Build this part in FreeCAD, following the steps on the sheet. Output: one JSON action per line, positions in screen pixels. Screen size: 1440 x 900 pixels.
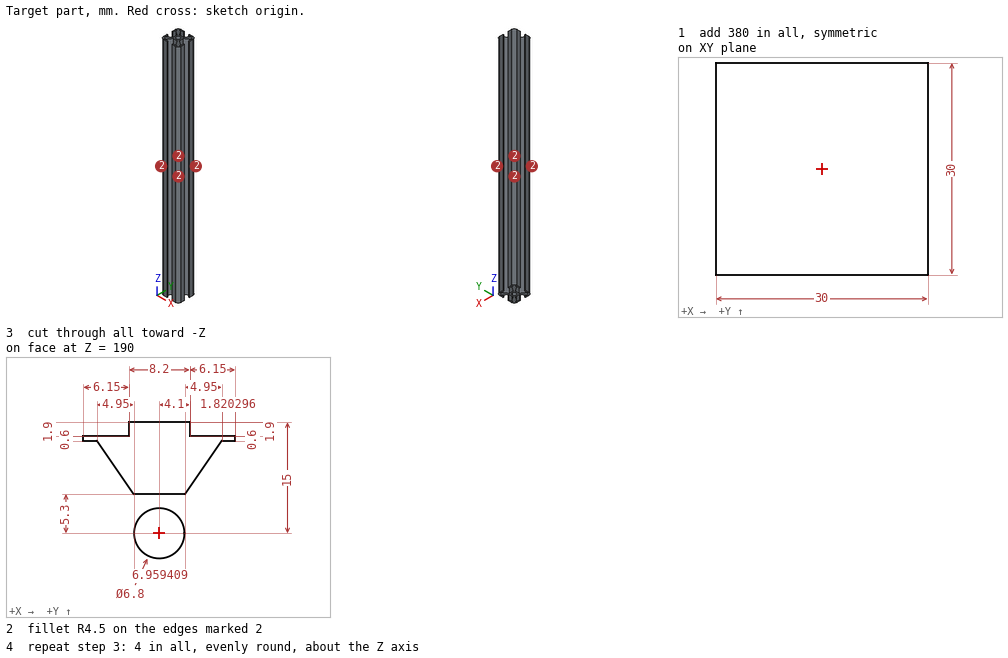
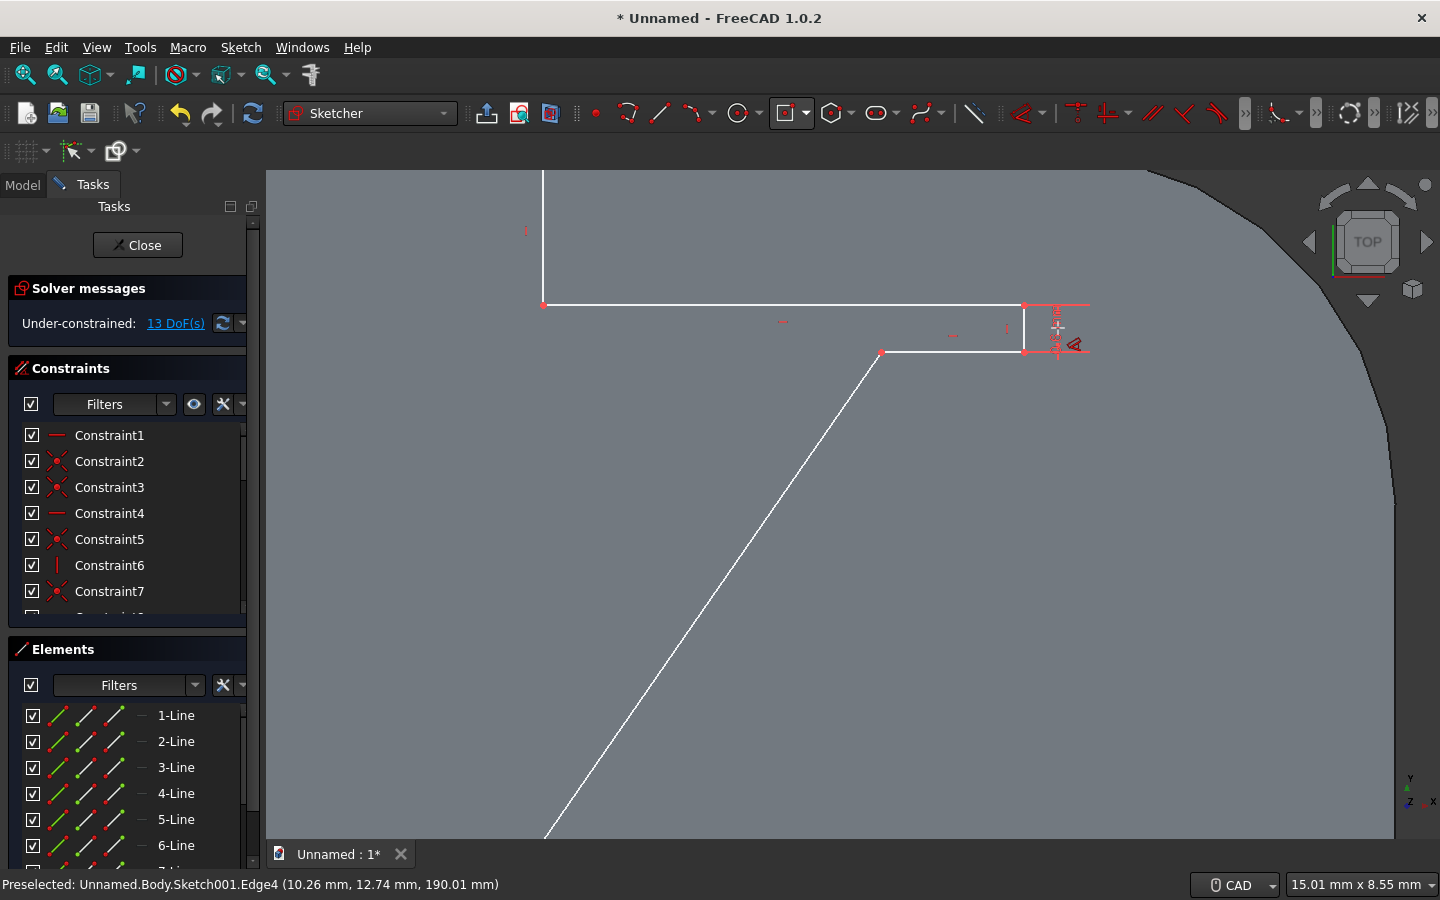
{"action": "left_click", "coordinate": [543, 260]}
{"action": "left_click", "coordinate": [577, 252]}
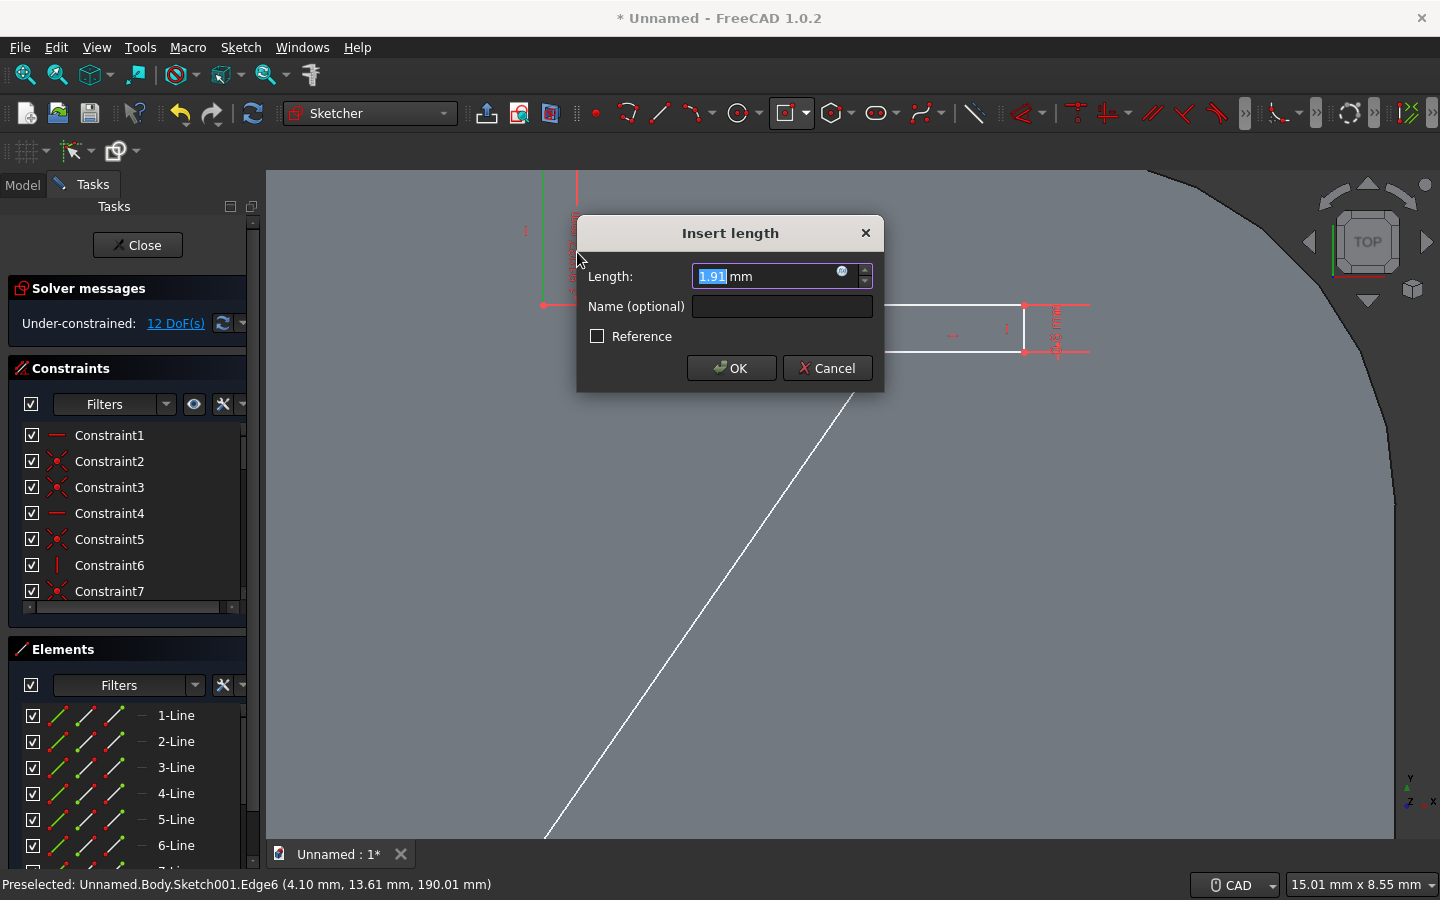
{"action": "type", "text": "1.9"}
{"action": "key", "text": "Return"}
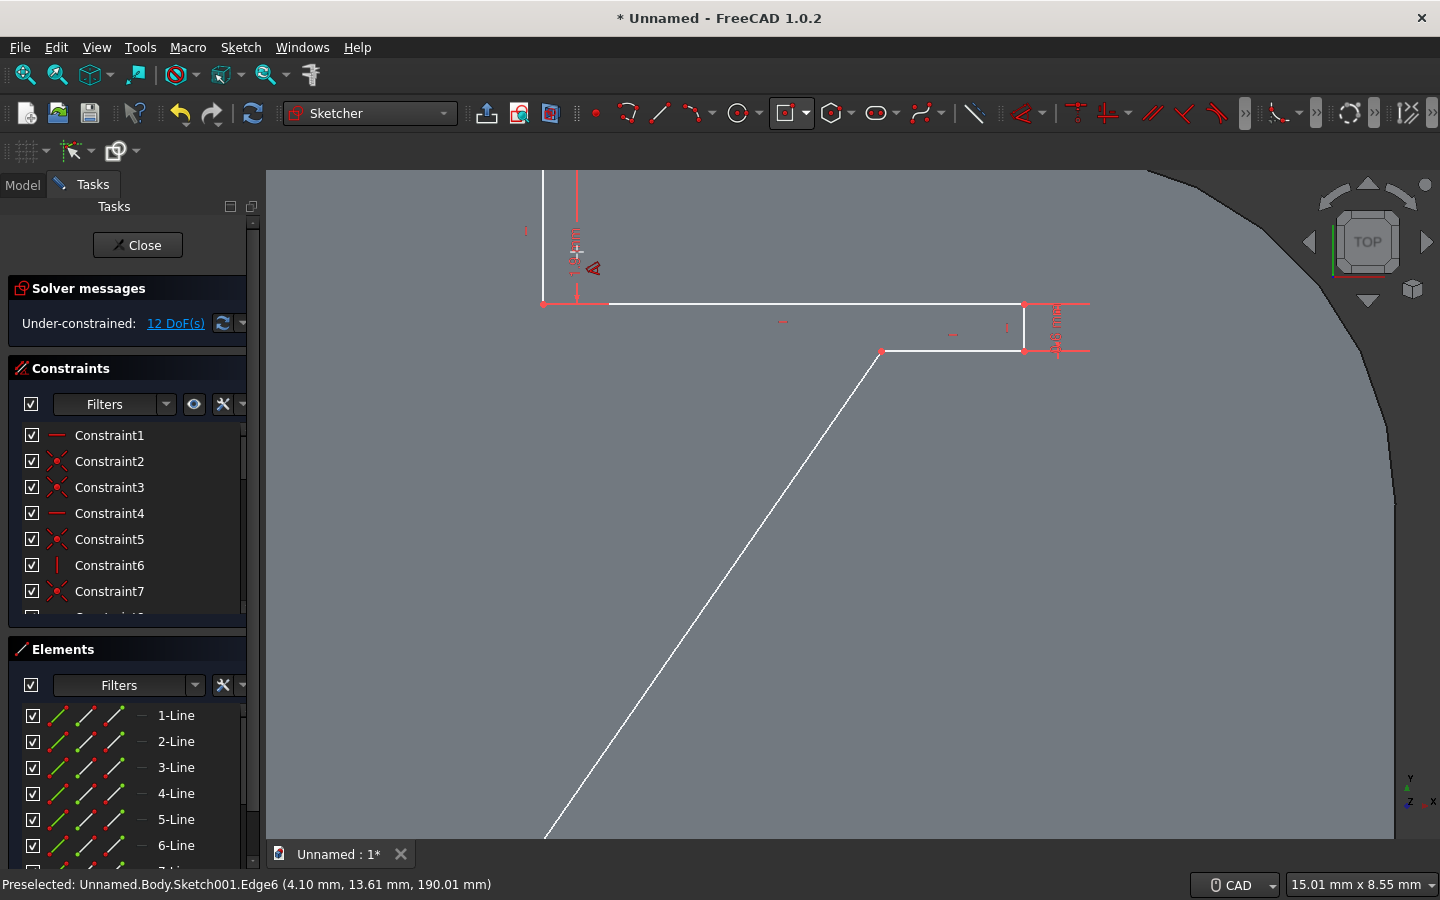
{"action": "scroll", "coordinate": [1027, 346], "scroll_direction": "down", "scroll_amount": 6}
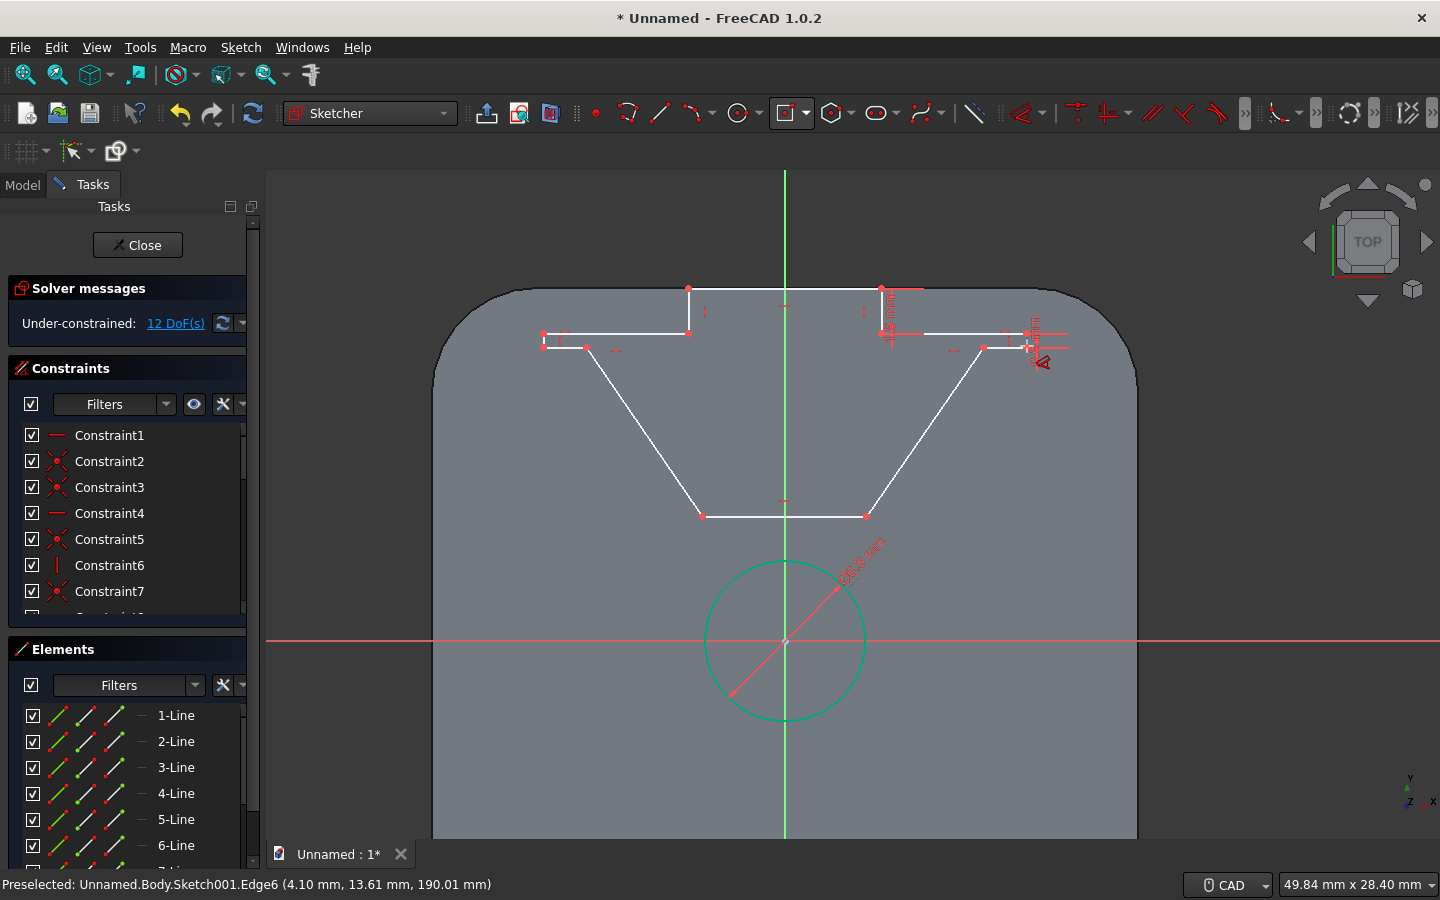
{"action": "left_click", "coordinate": [824, 289]}
{"action": "left_click", "coordinate": [741, 255]}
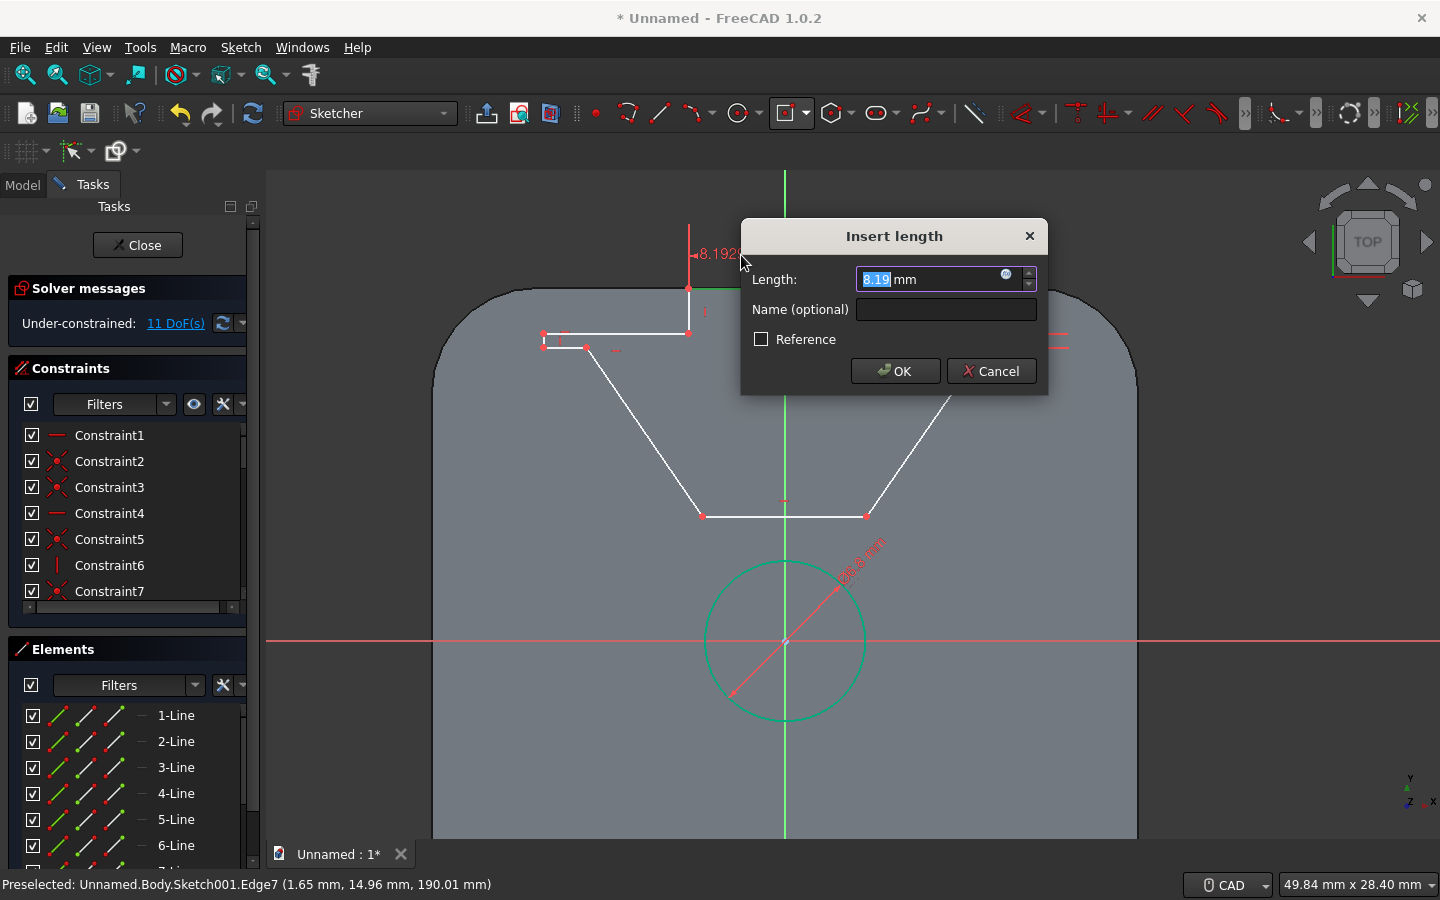
{"action": "type", "text": "8.2"}
{"action": "key", "text": "Return"}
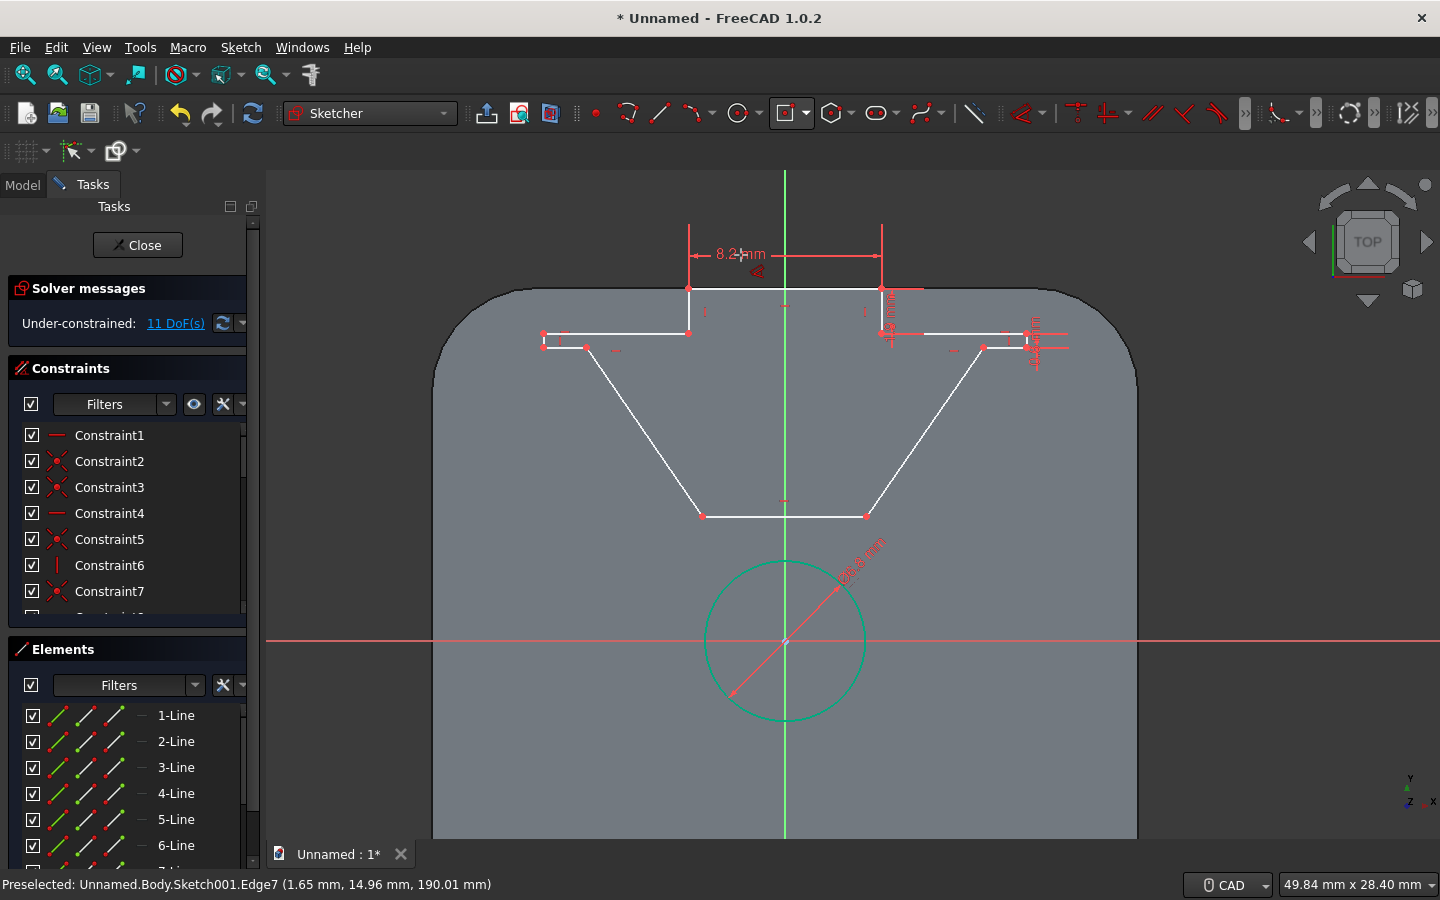
{"action": "left_click", "coordinate": [689, 302]}
{"action": "left_click", "coordinate": [655, 311]}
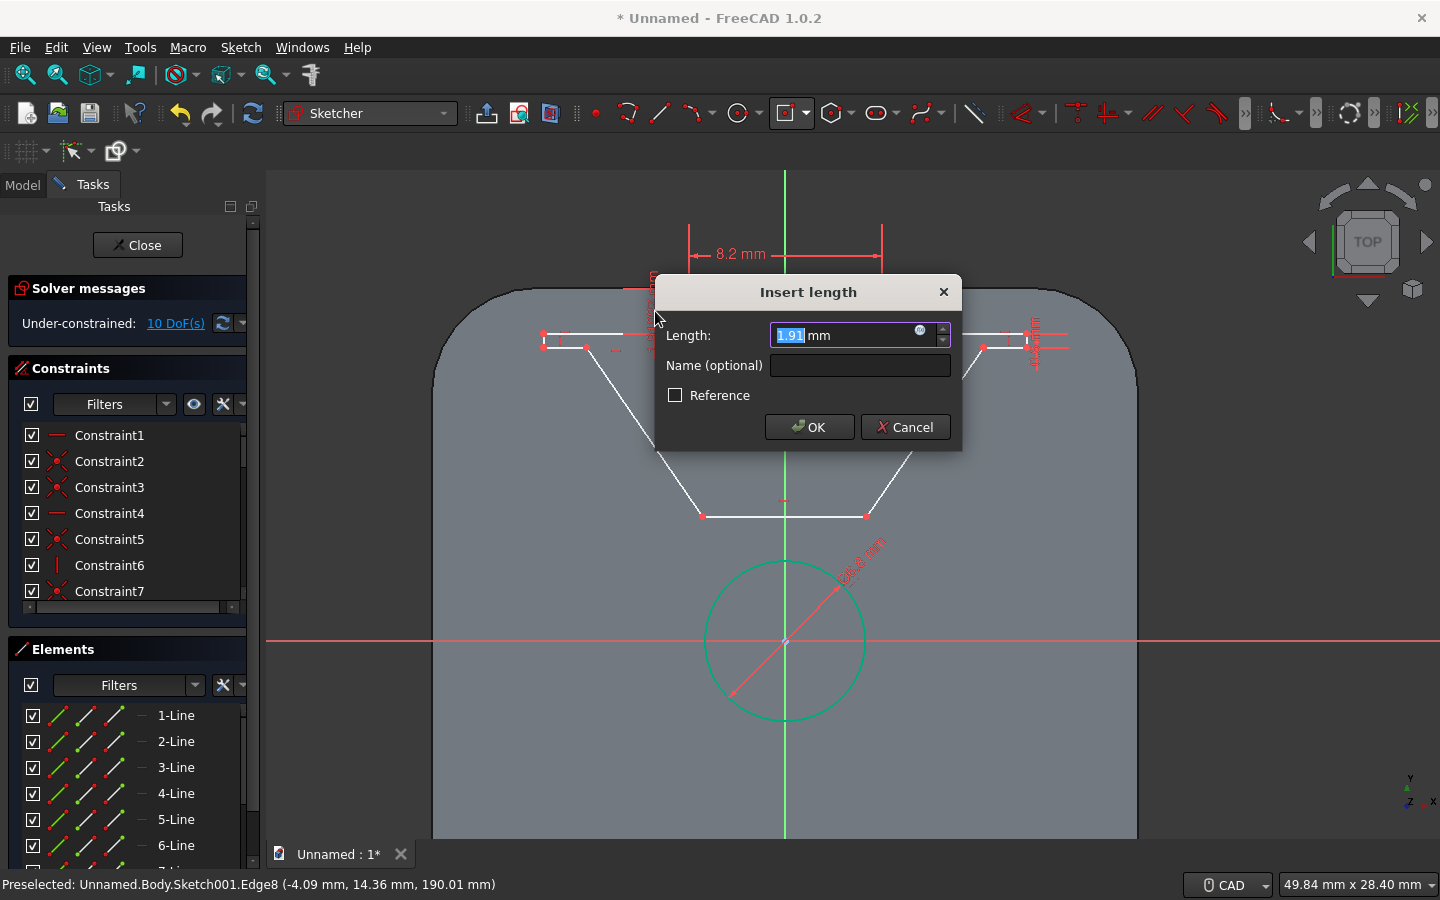
{"action": "type", "text": "1.9"}
{"action": "key", "text": "Return"}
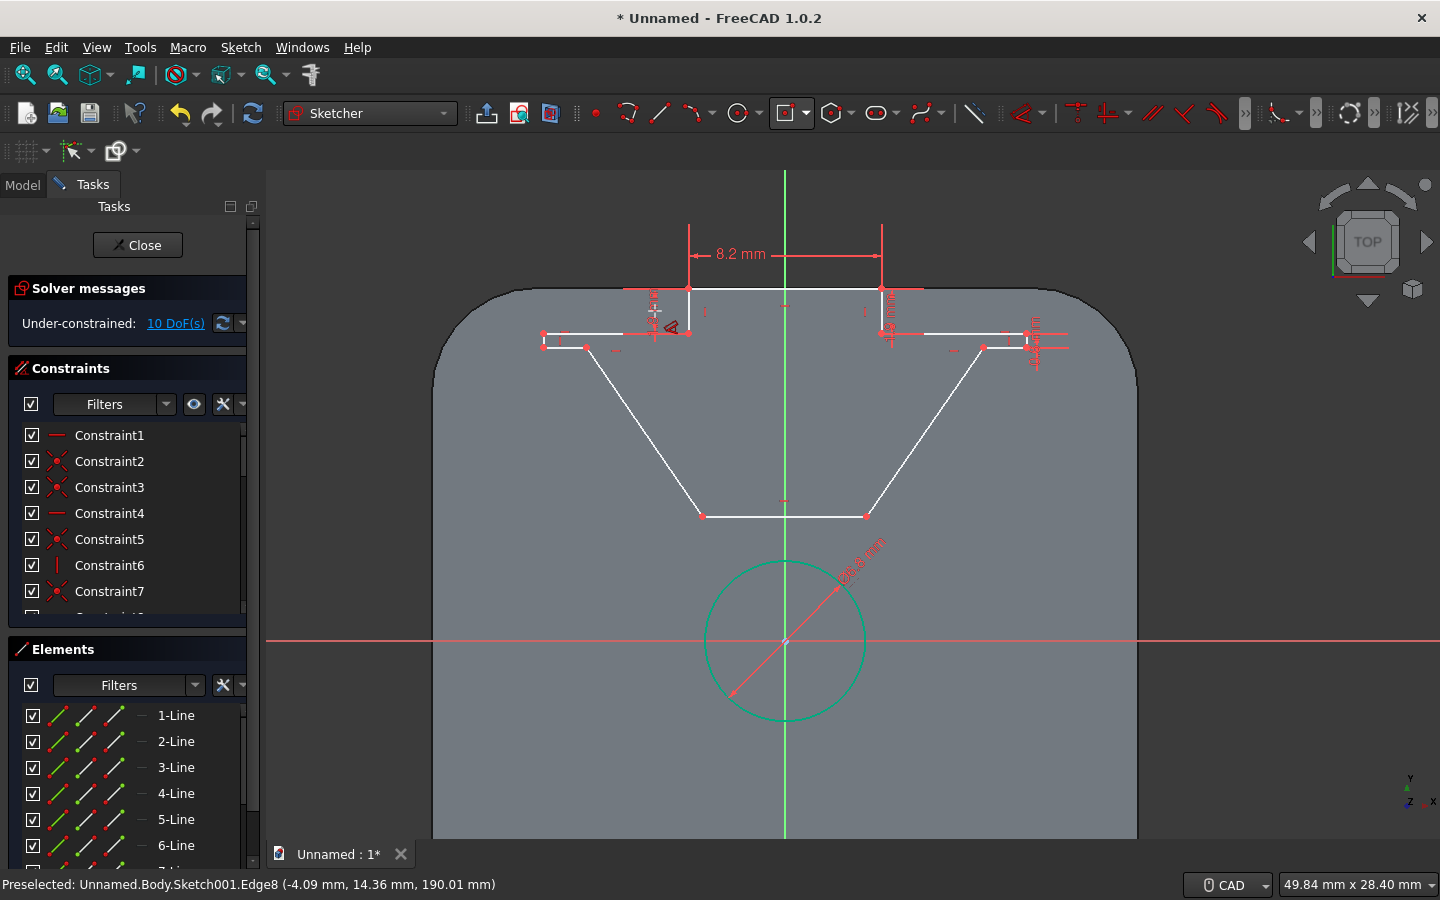
{"action": "scroll", "coordinate": [544, 341], "scroll_direction": "up", "scroll_amount": 6}